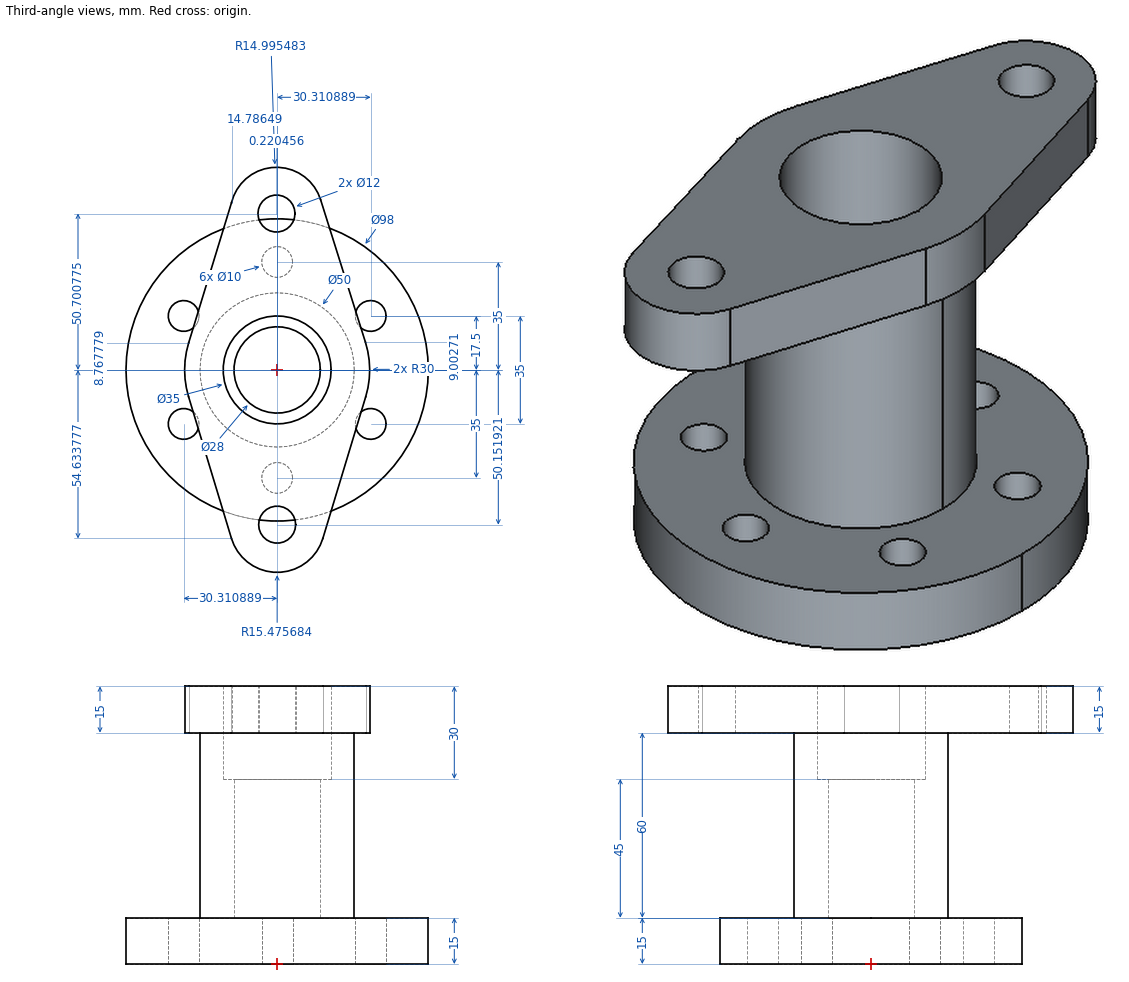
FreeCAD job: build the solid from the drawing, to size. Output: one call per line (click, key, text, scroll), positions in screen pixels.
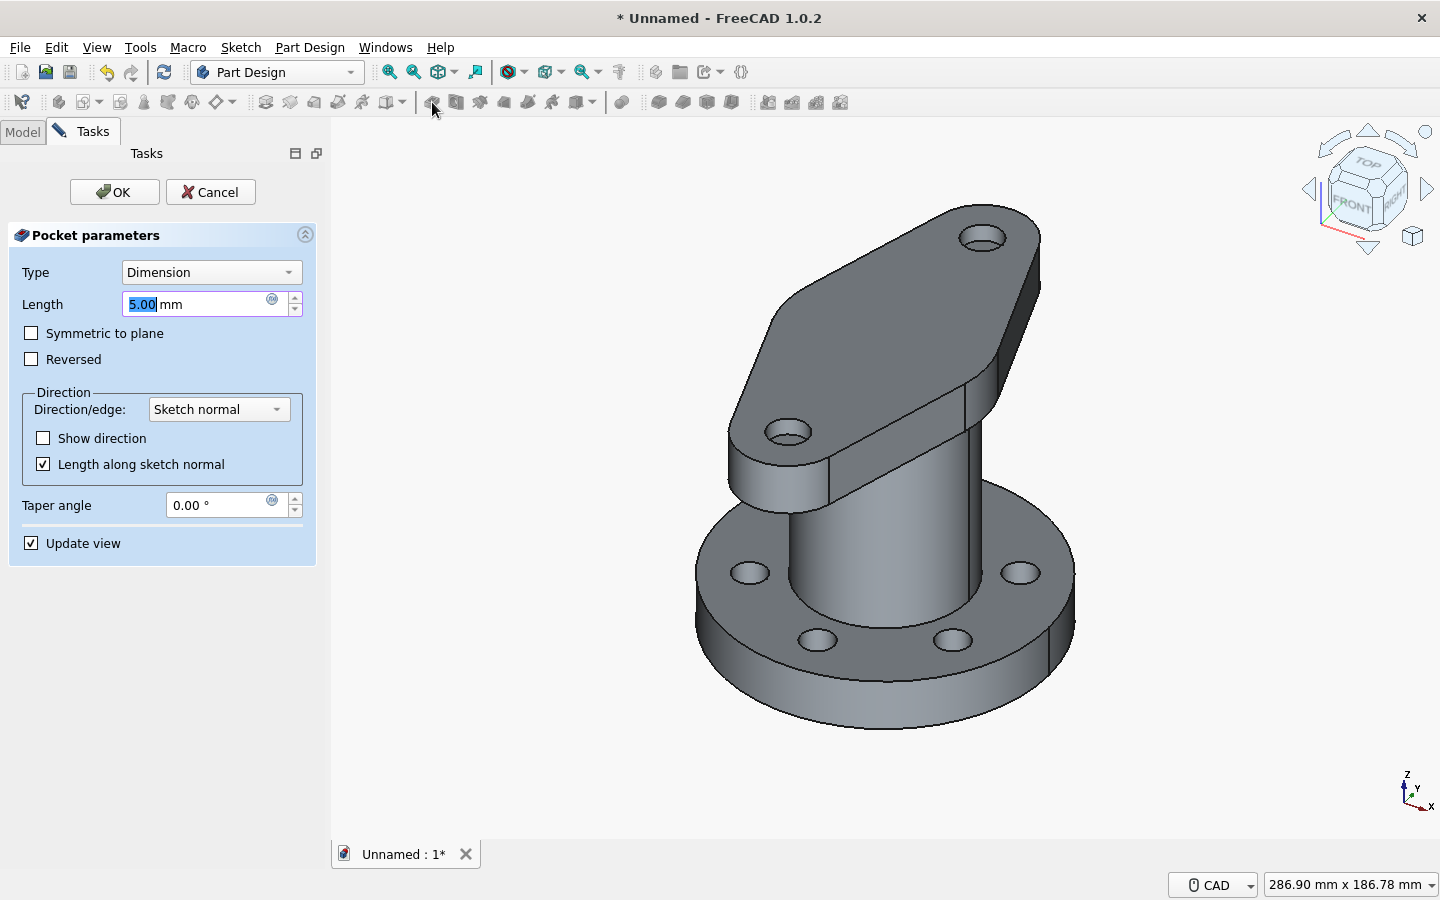
text(15)
key(Tab)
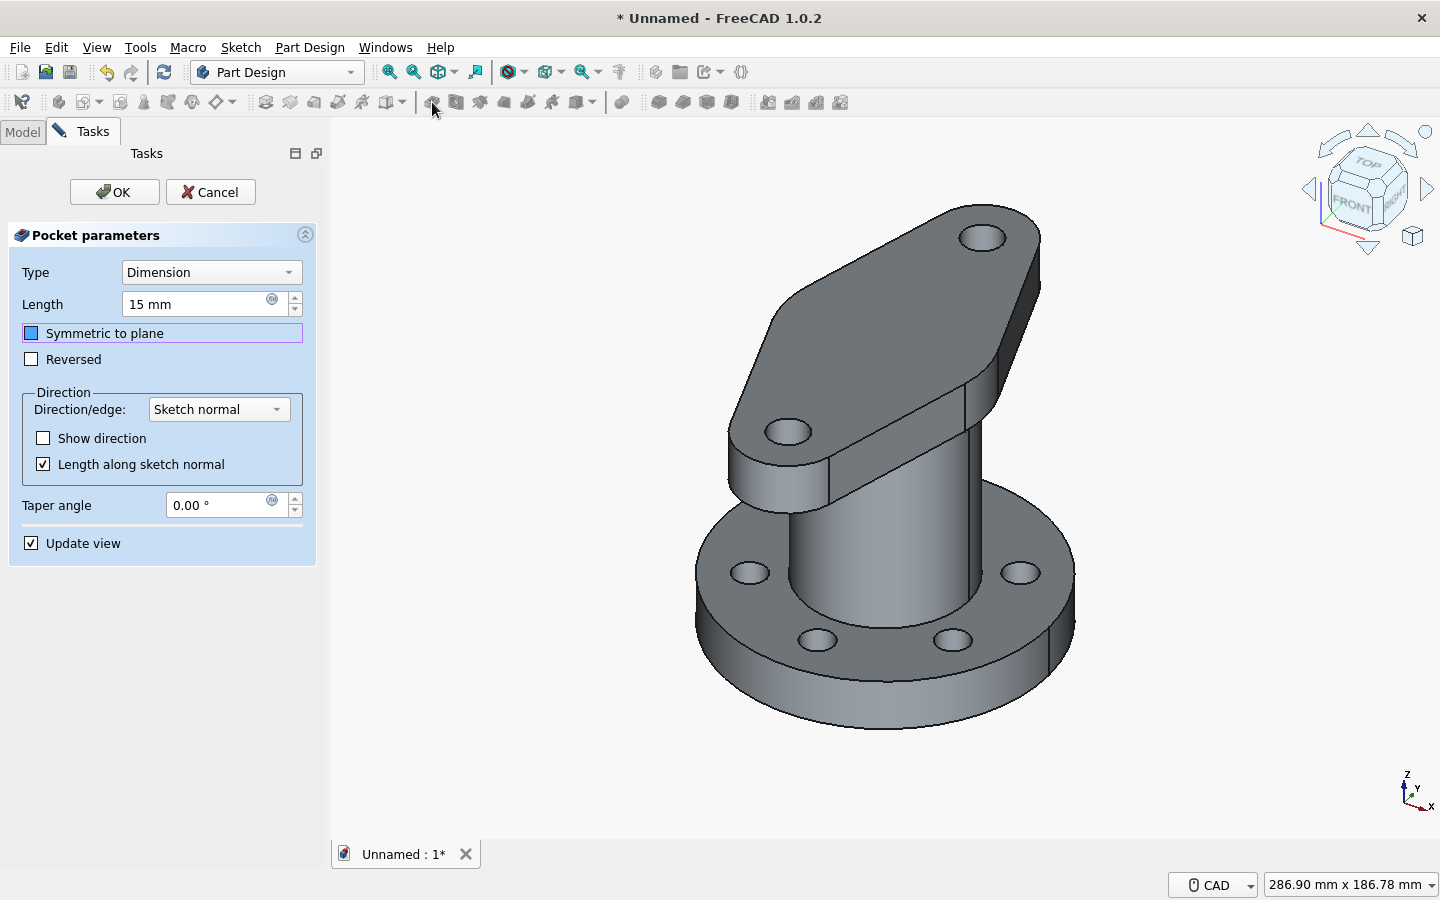
click(115, 192)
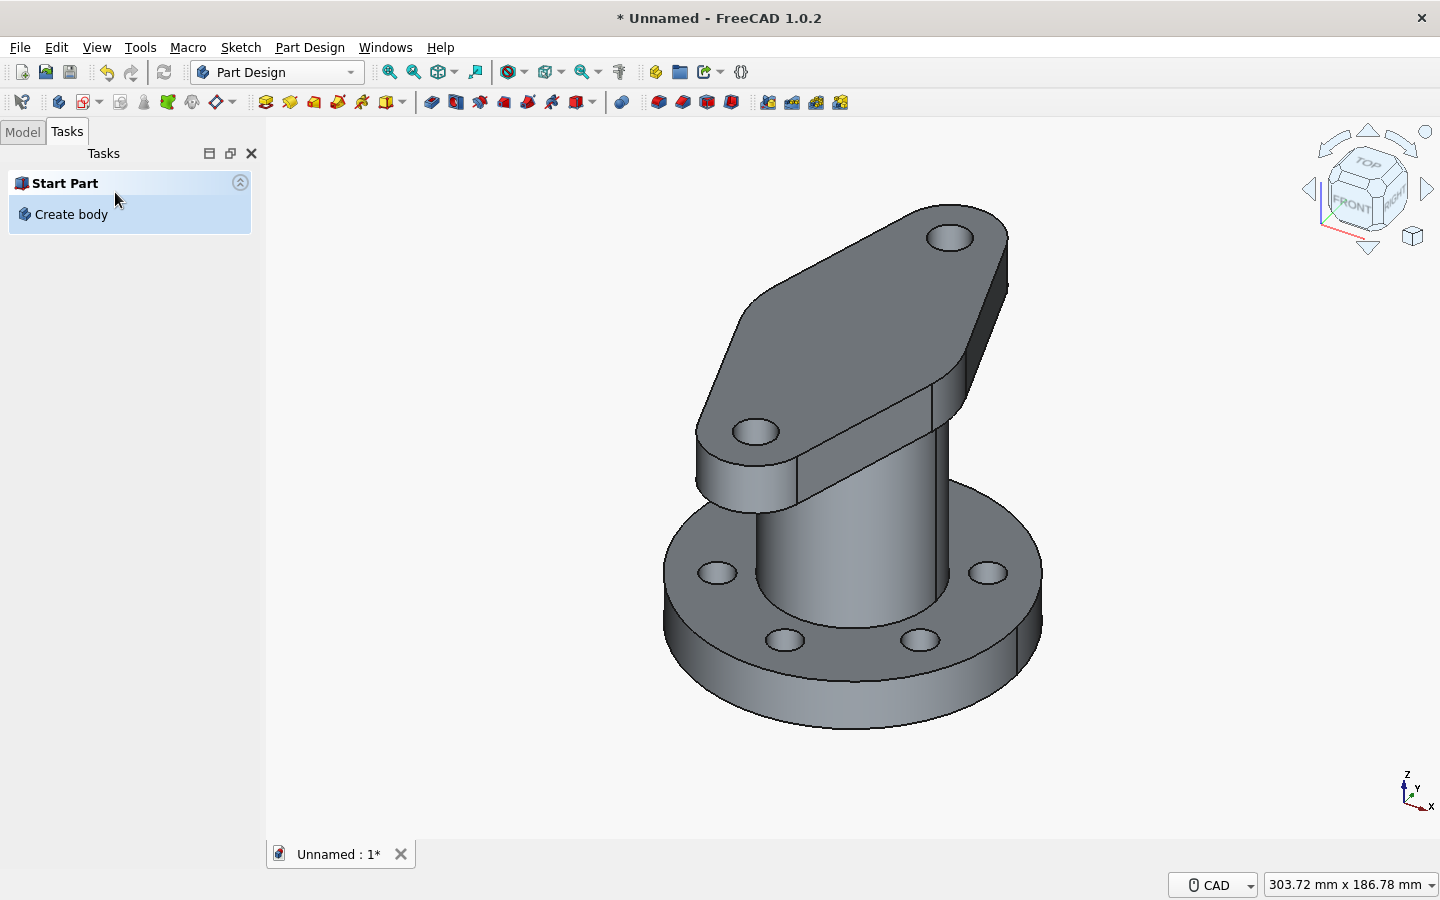
click(853, 335)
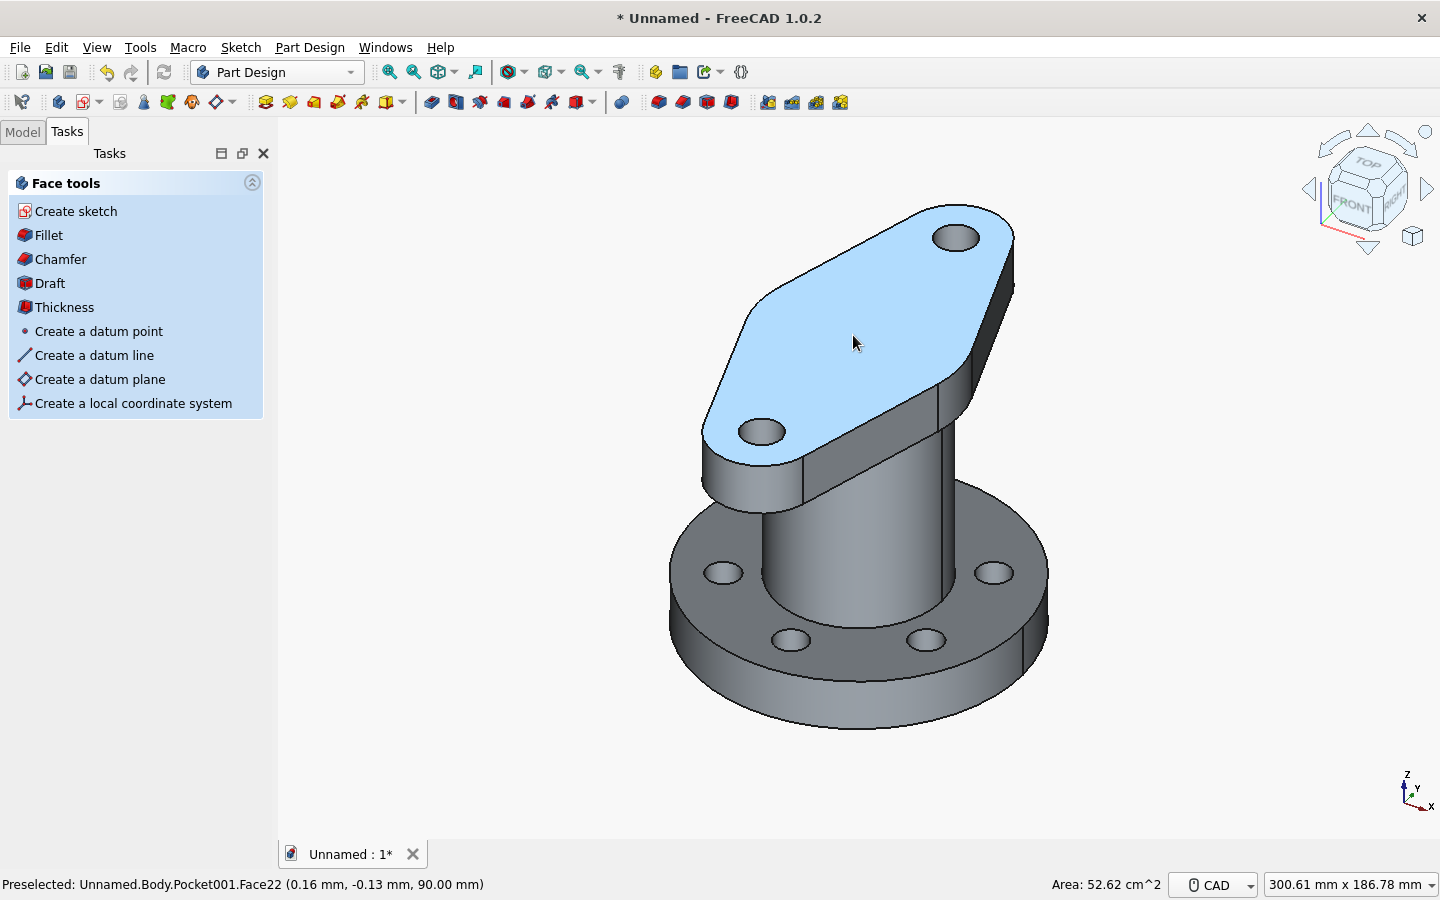
click(84, 102)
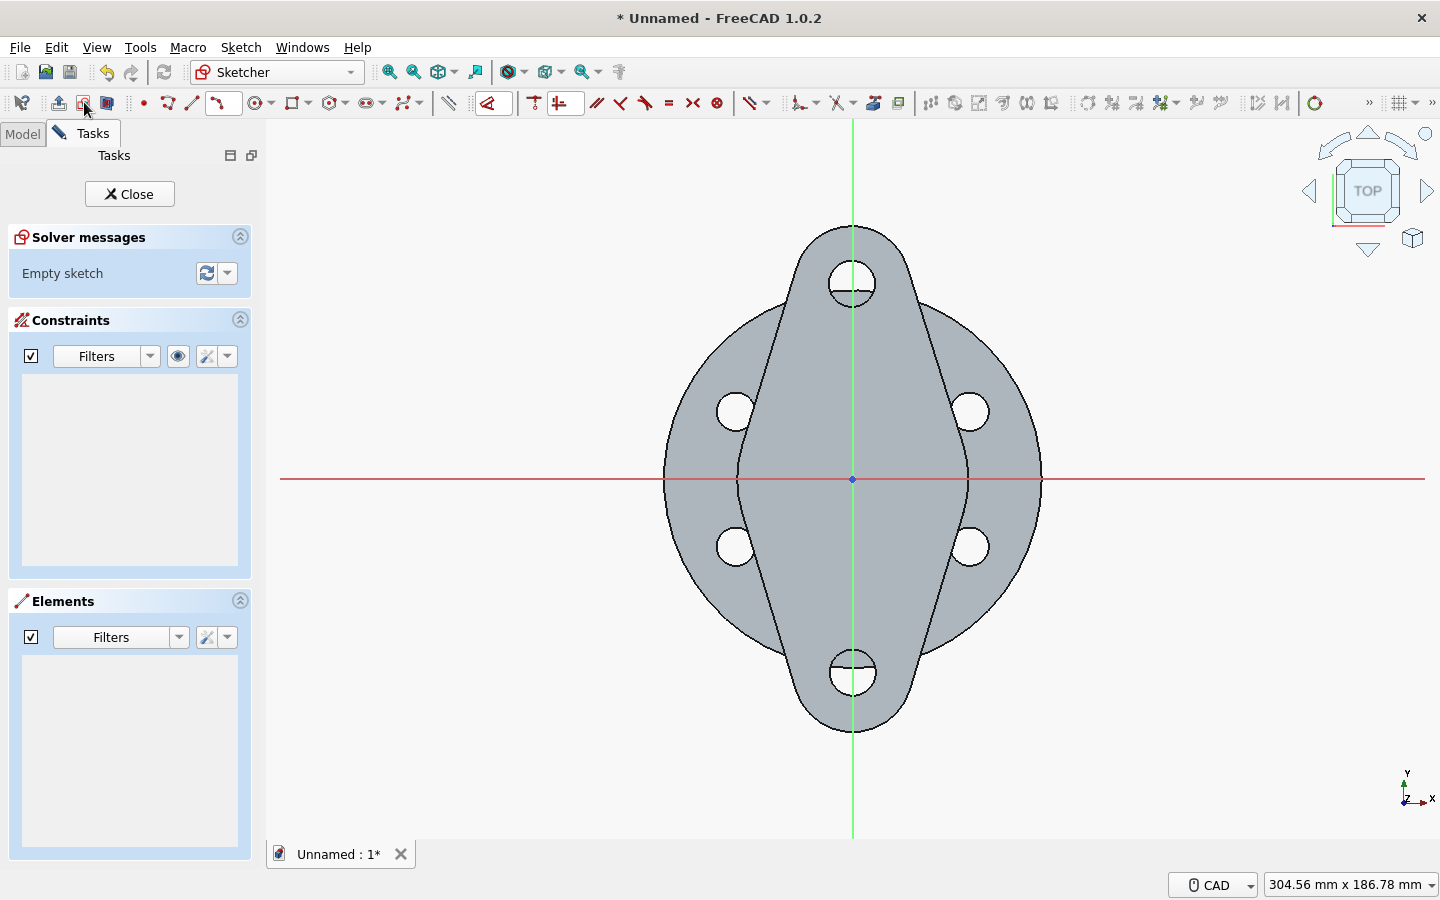
scroll(882, 479, up, 6)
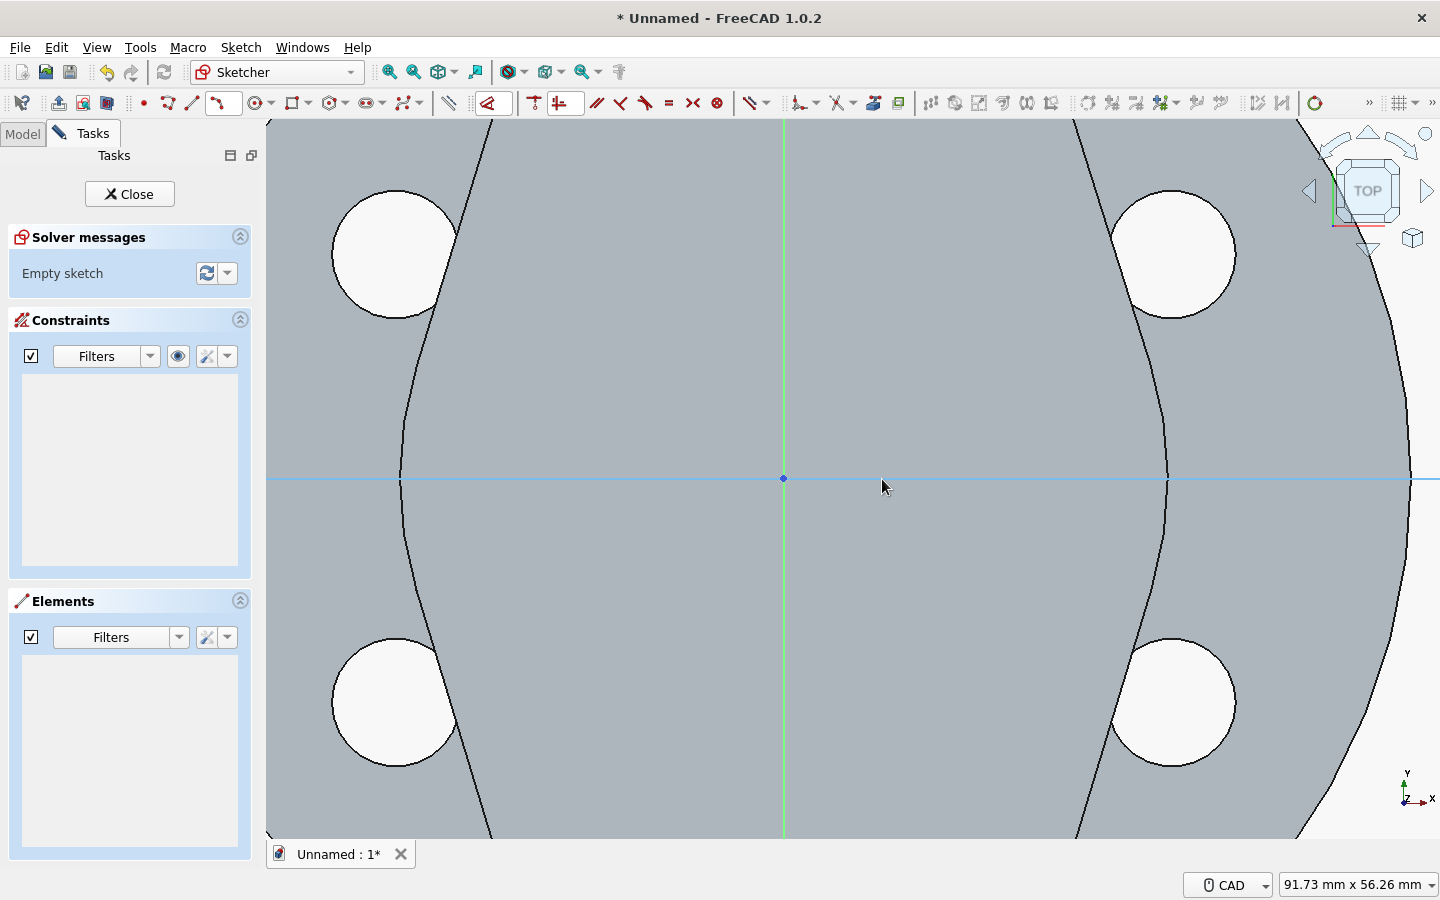
key(g)
key(c)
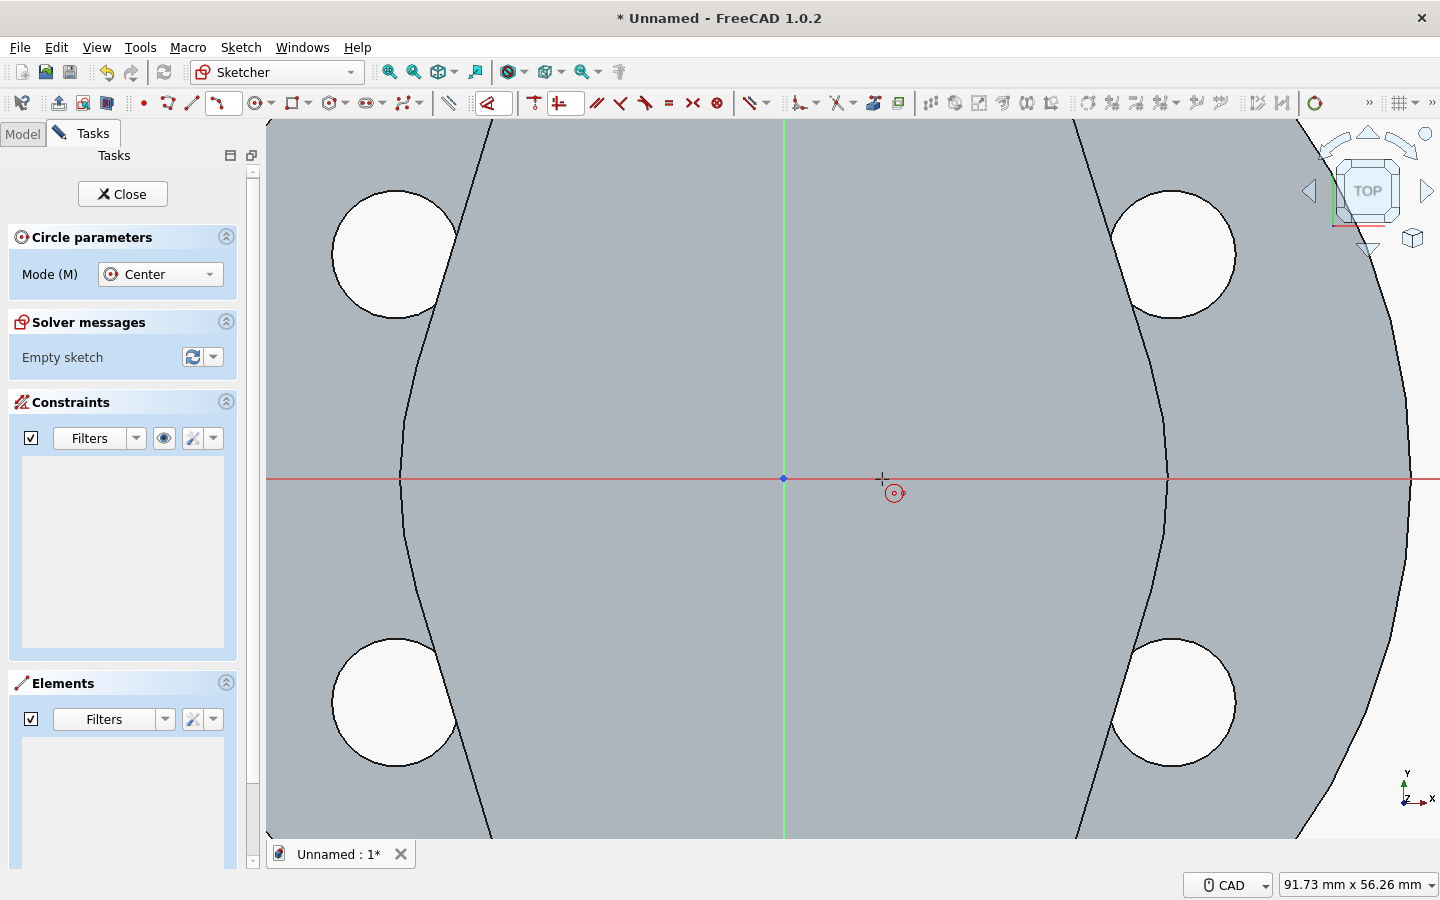
click(784, 479)
click(942, 320)
key(Escape)